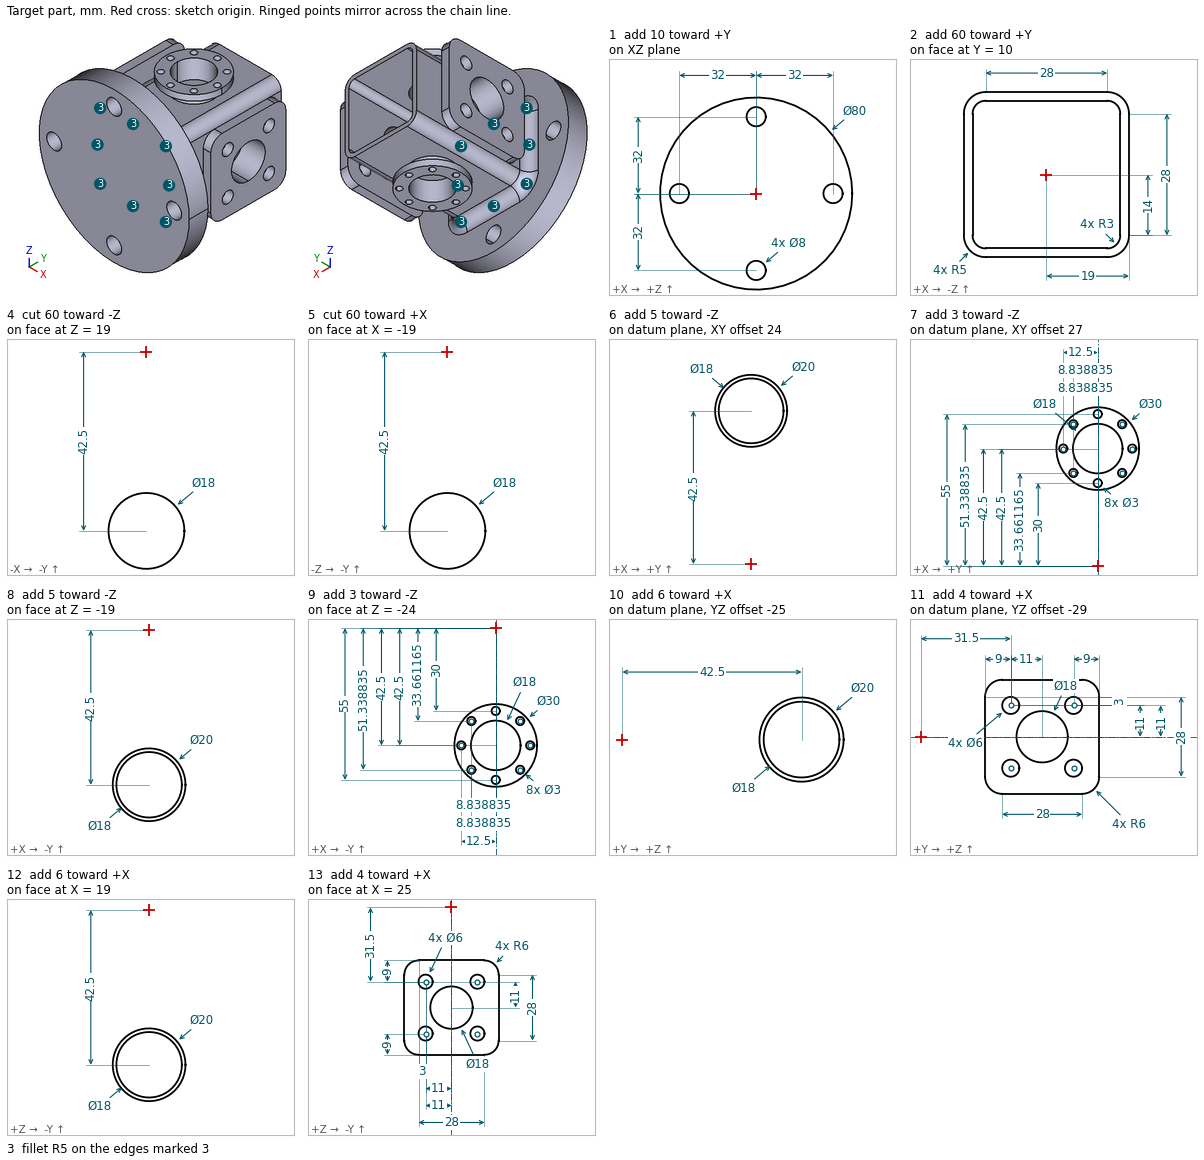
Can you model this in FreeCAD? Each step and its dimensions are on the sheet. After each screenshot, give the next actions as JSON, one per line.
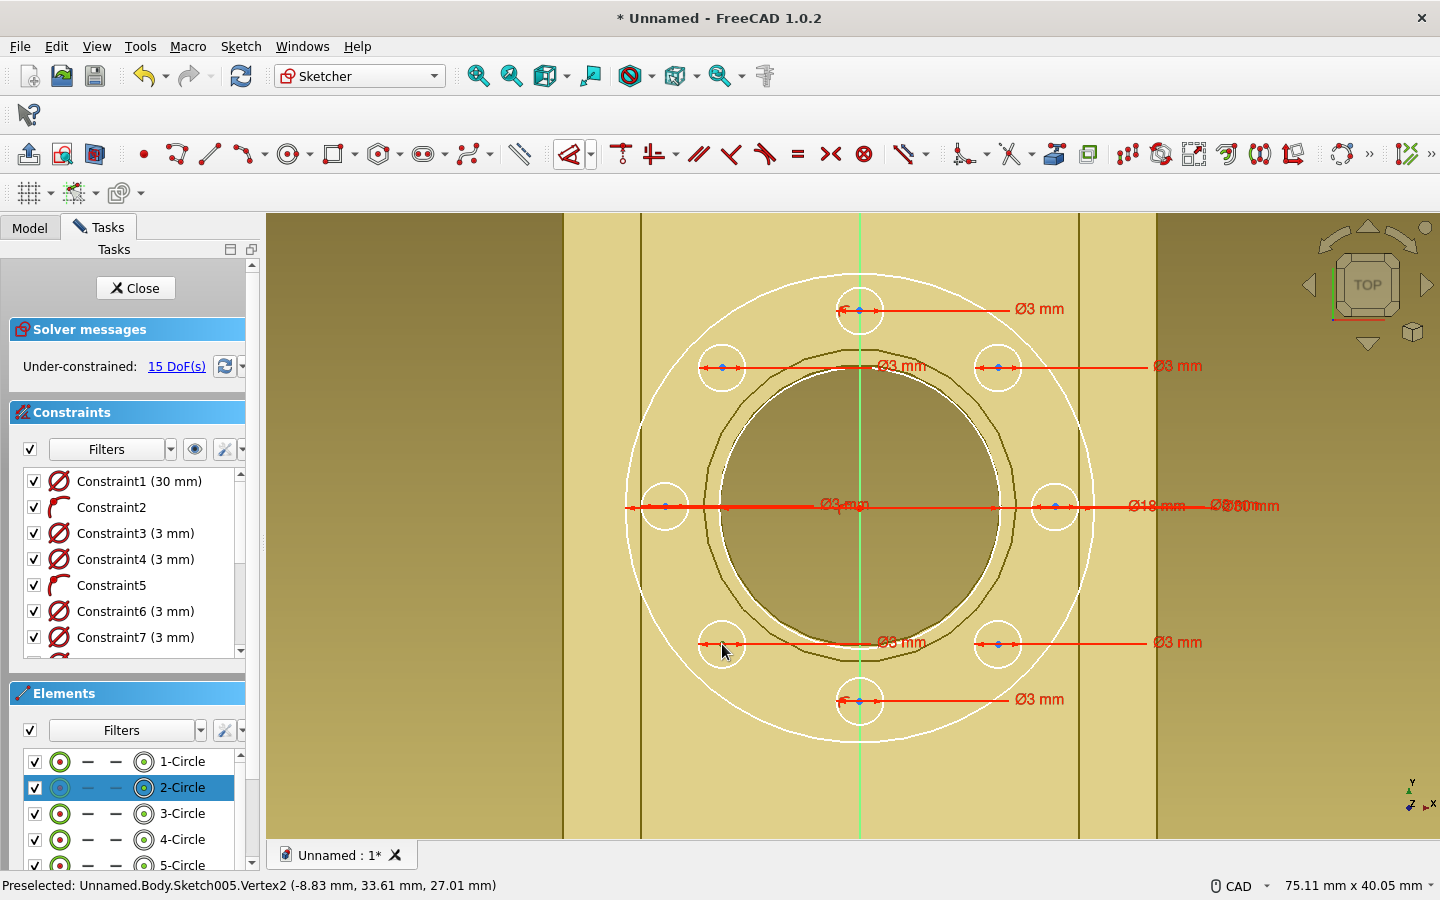
{"action": "left_click", "coordinate": [998, 644]}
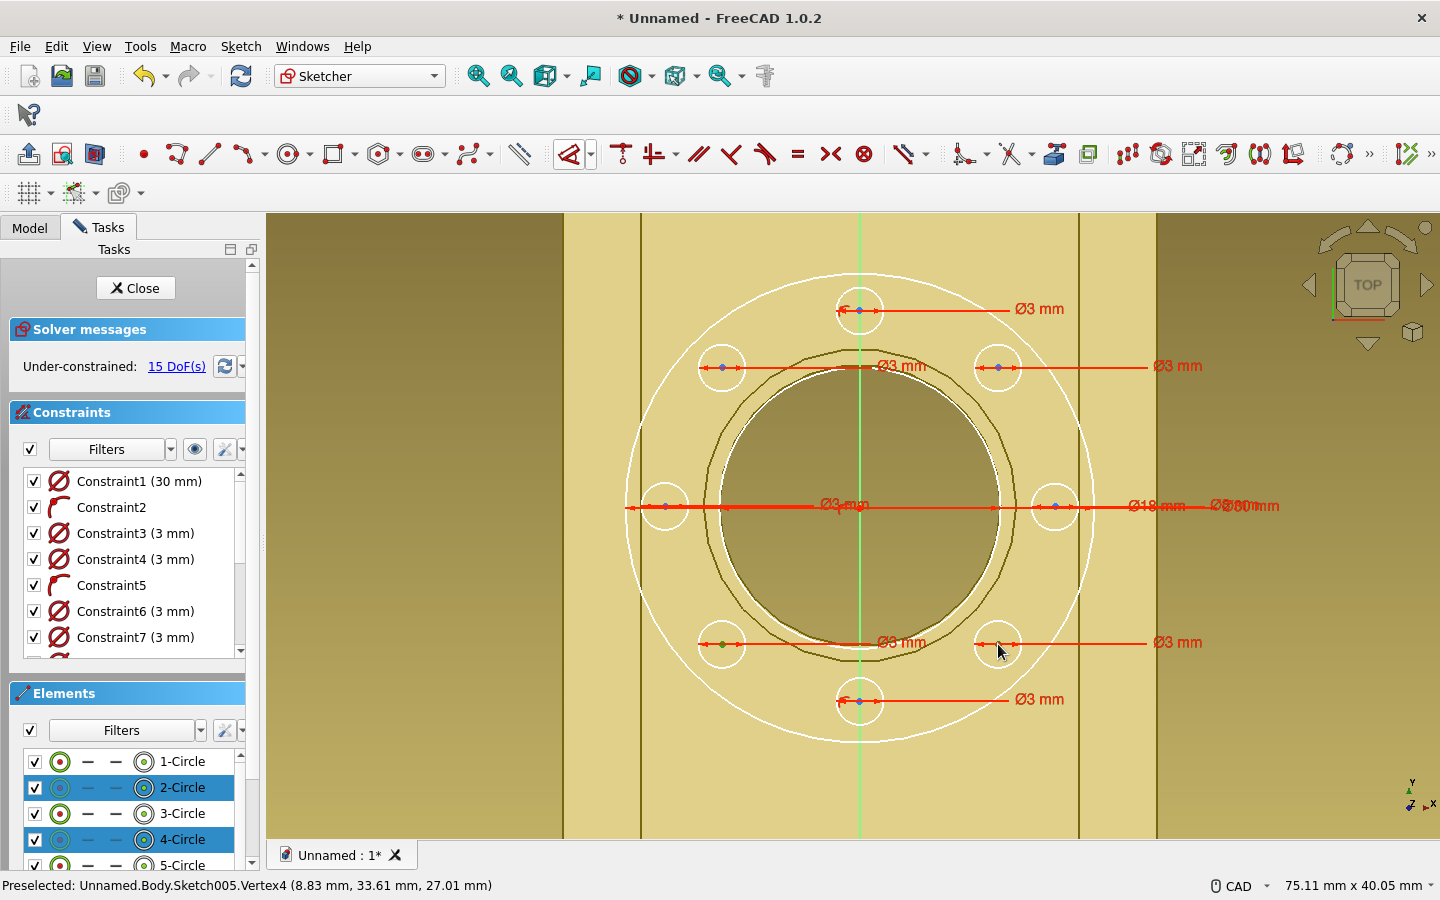
{"action": "left_click", "coordinate": [860, 607]}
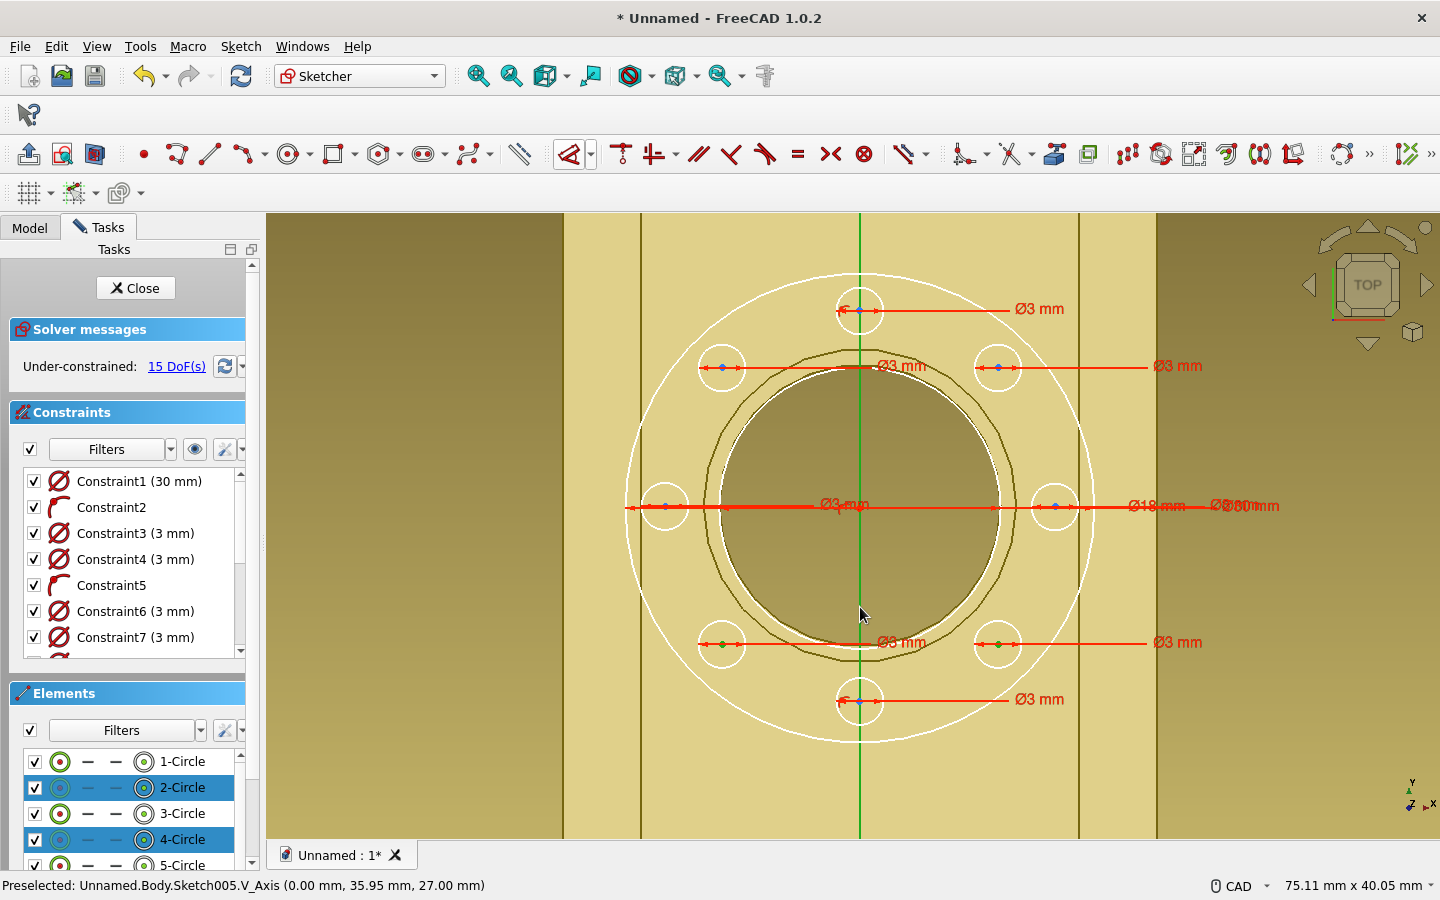
{"action": "key", "text": "s"}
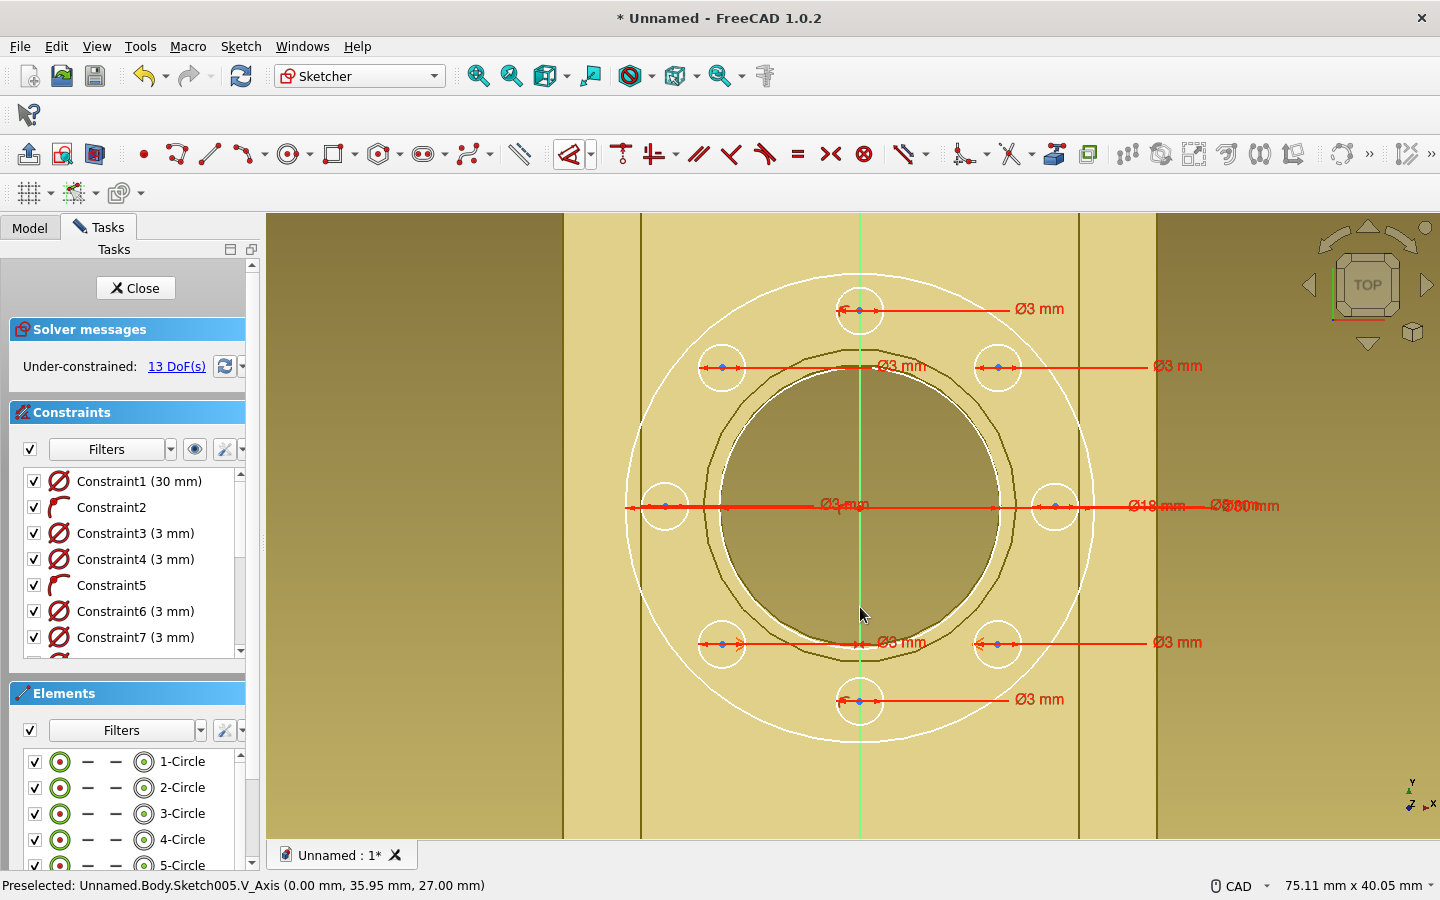
{"action": "left_click", "coordinate": [665, 506]}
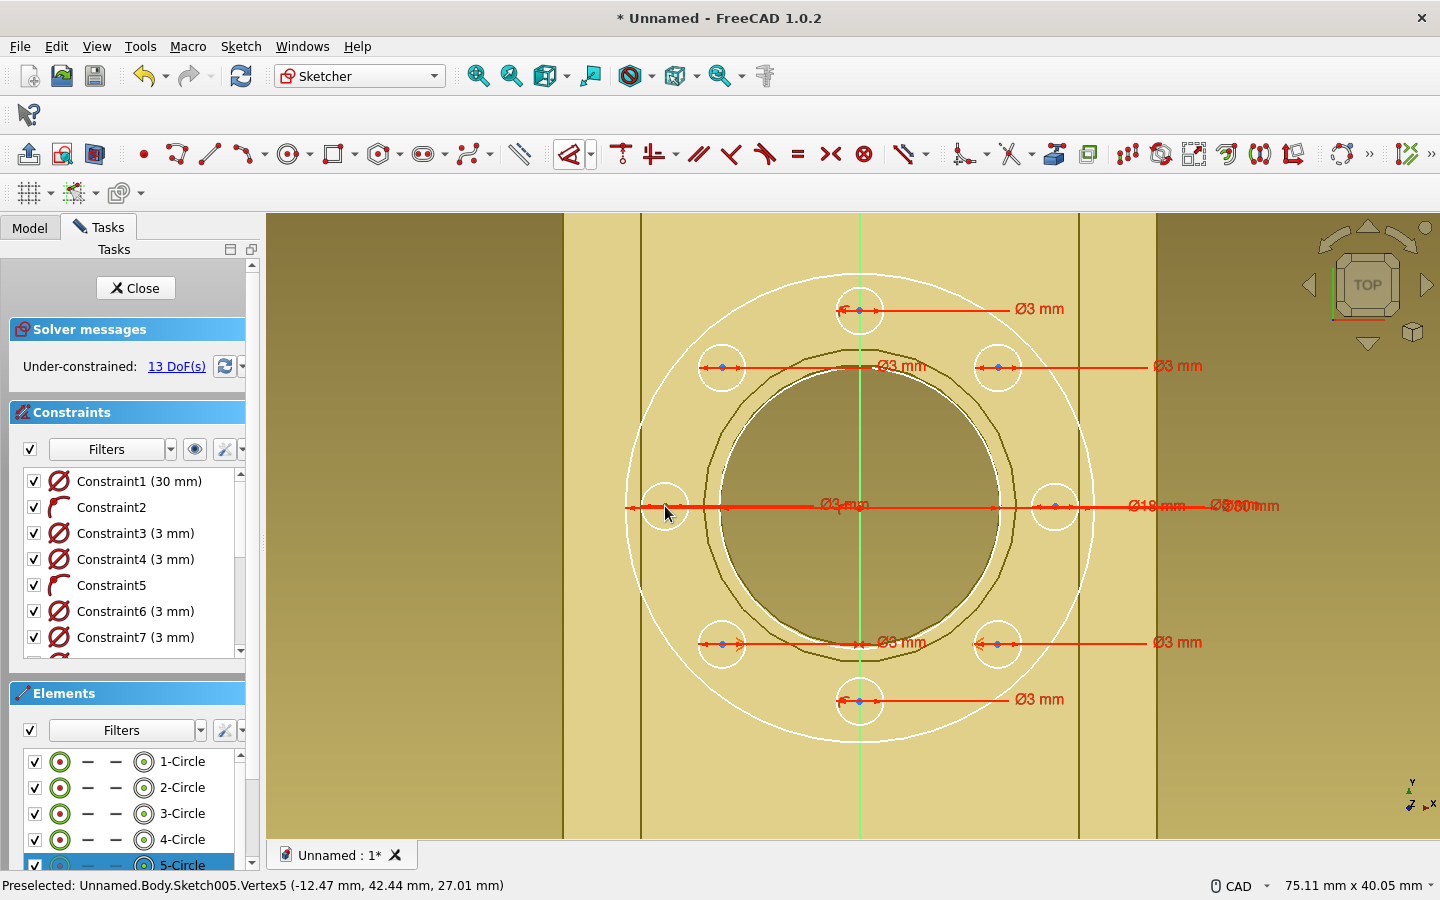
{"action": "left_click", "coordinate": [1055, 507]}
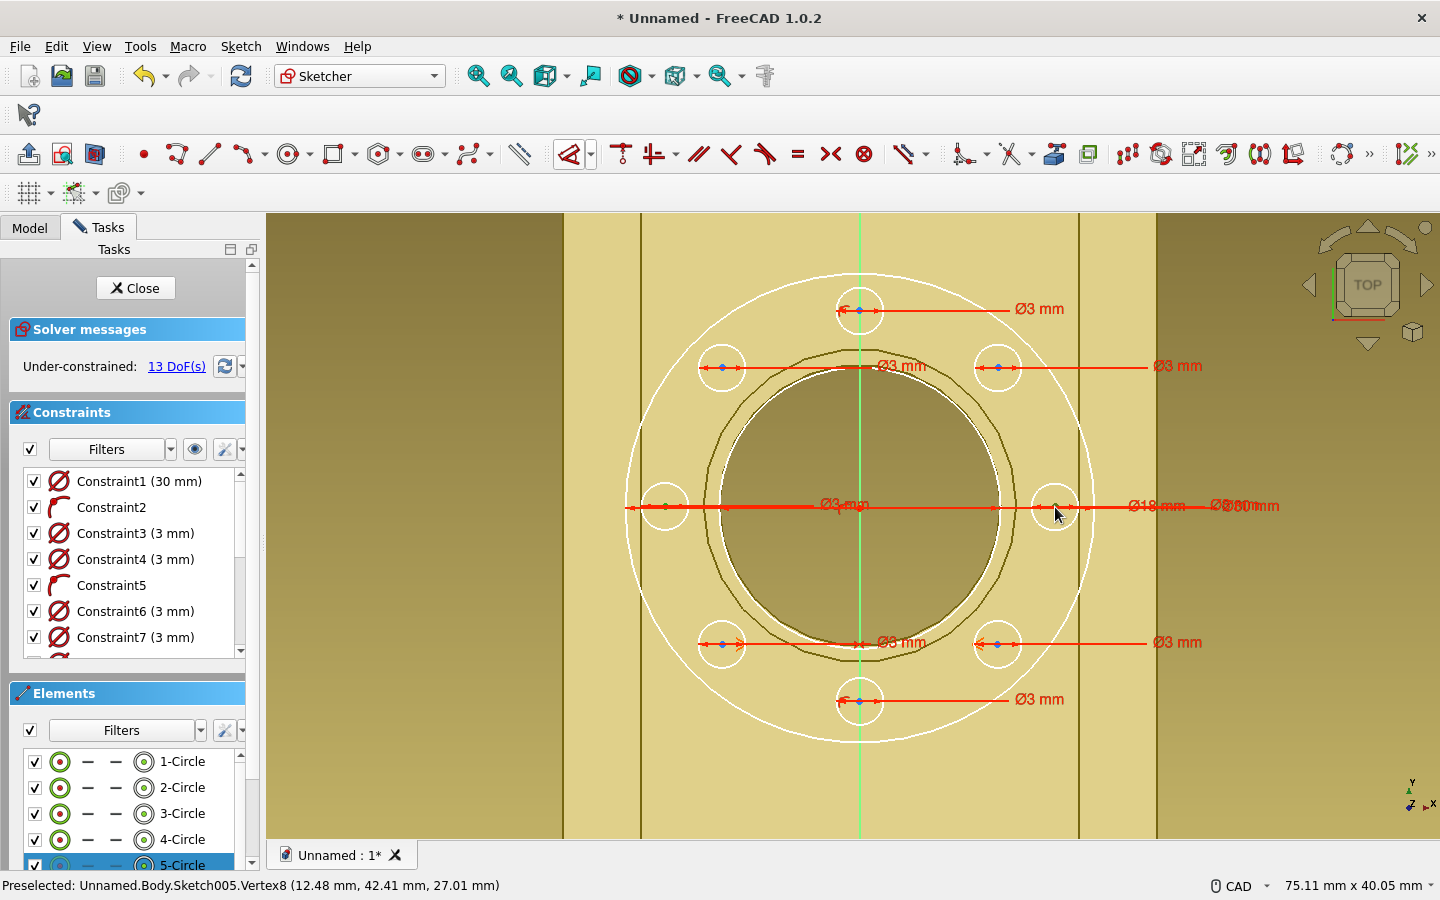
{"action": "left_click", "coordinate": [860, 607]}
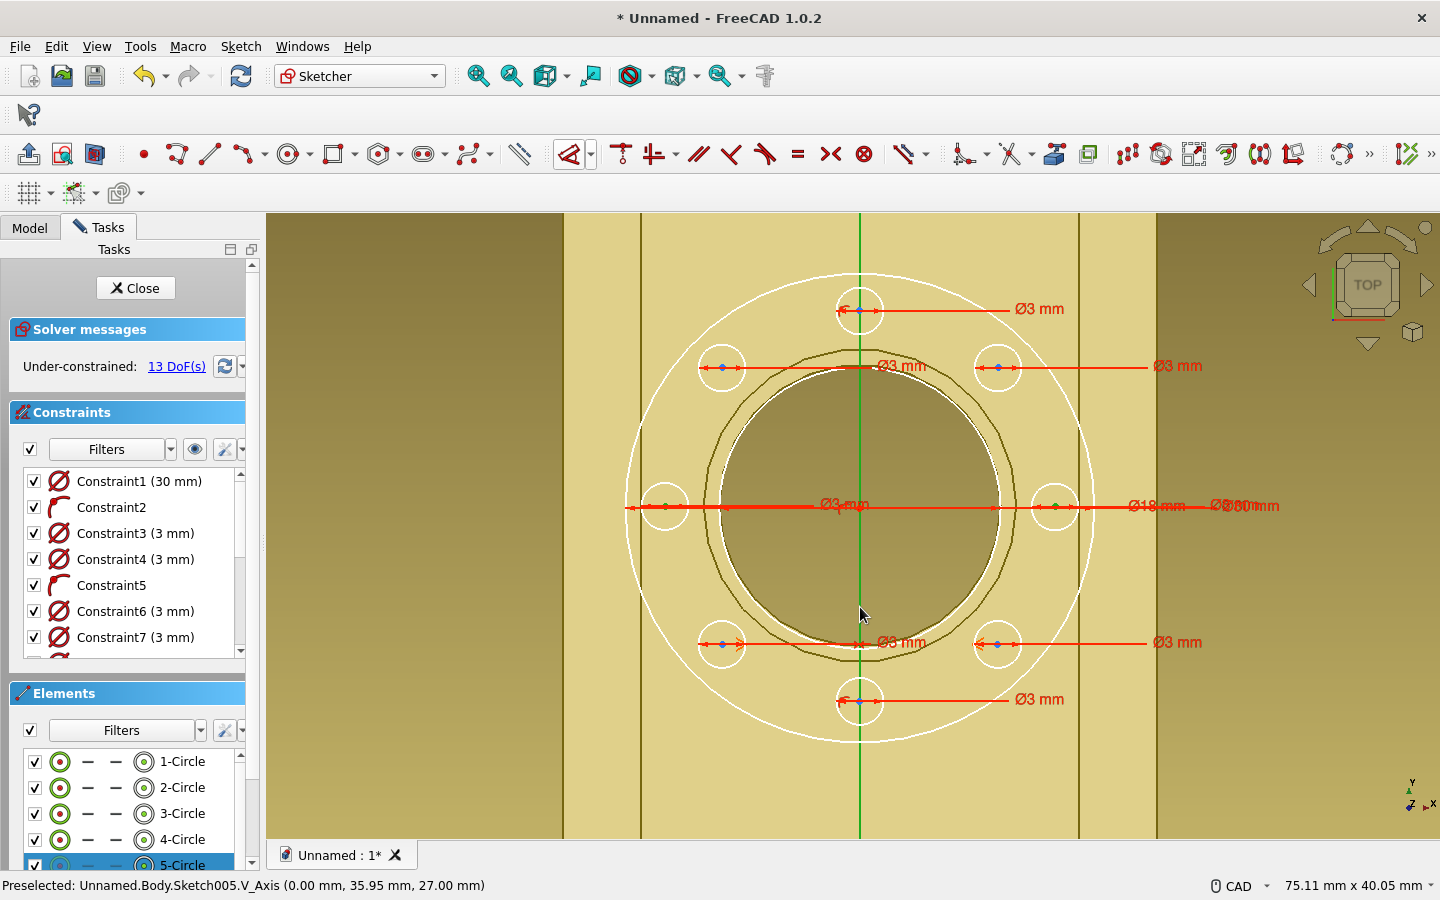
{"action": "key", "text": "s"}